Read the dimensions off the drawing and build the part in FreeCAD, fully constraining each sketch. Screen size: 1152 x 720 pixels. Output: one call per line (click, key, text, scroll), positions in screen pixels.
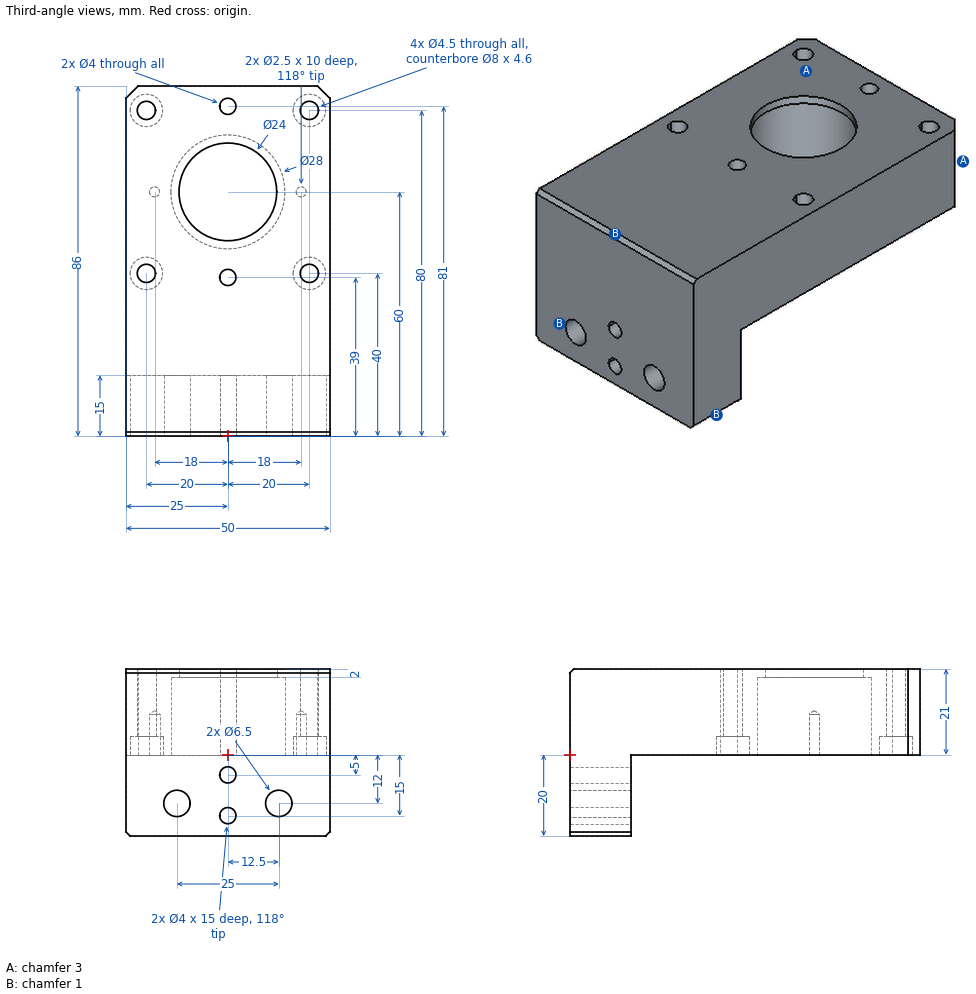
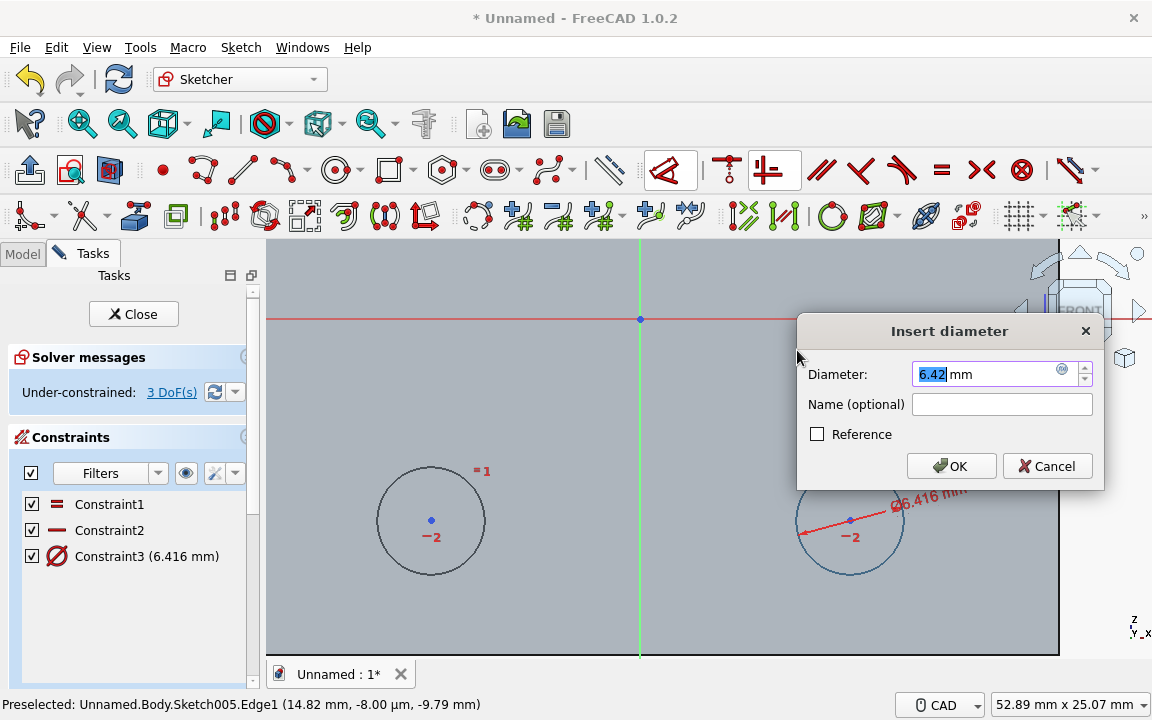
text(6.5)
key(Return)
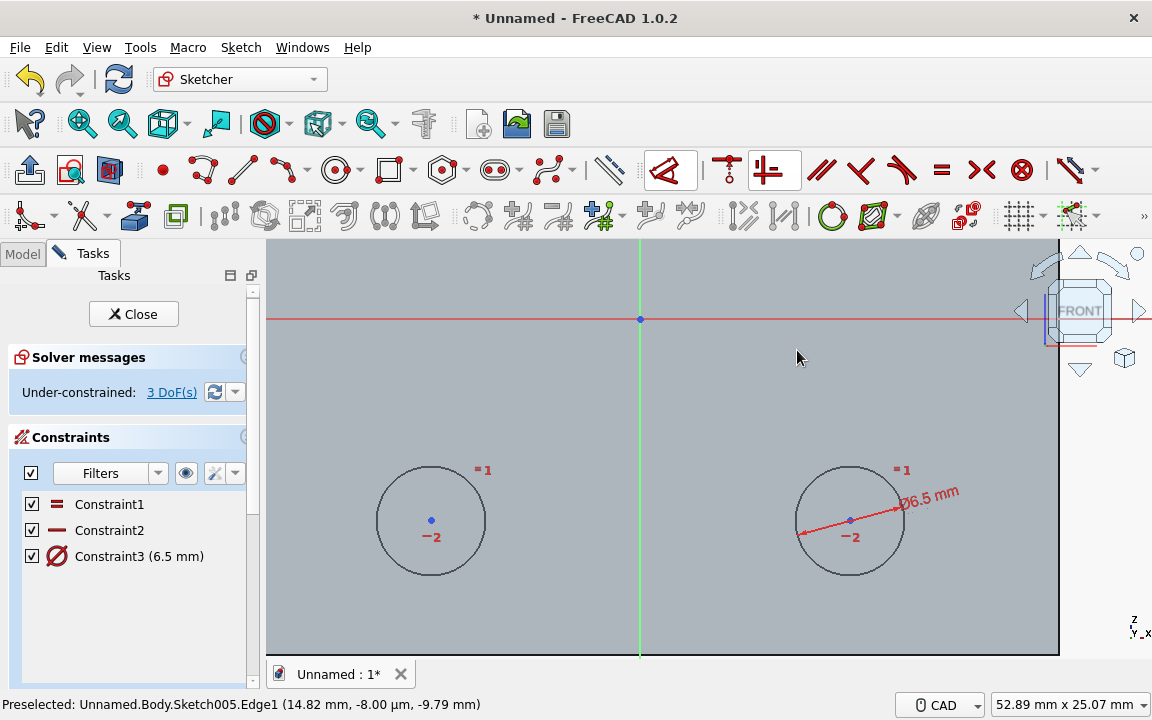
click(850, 521)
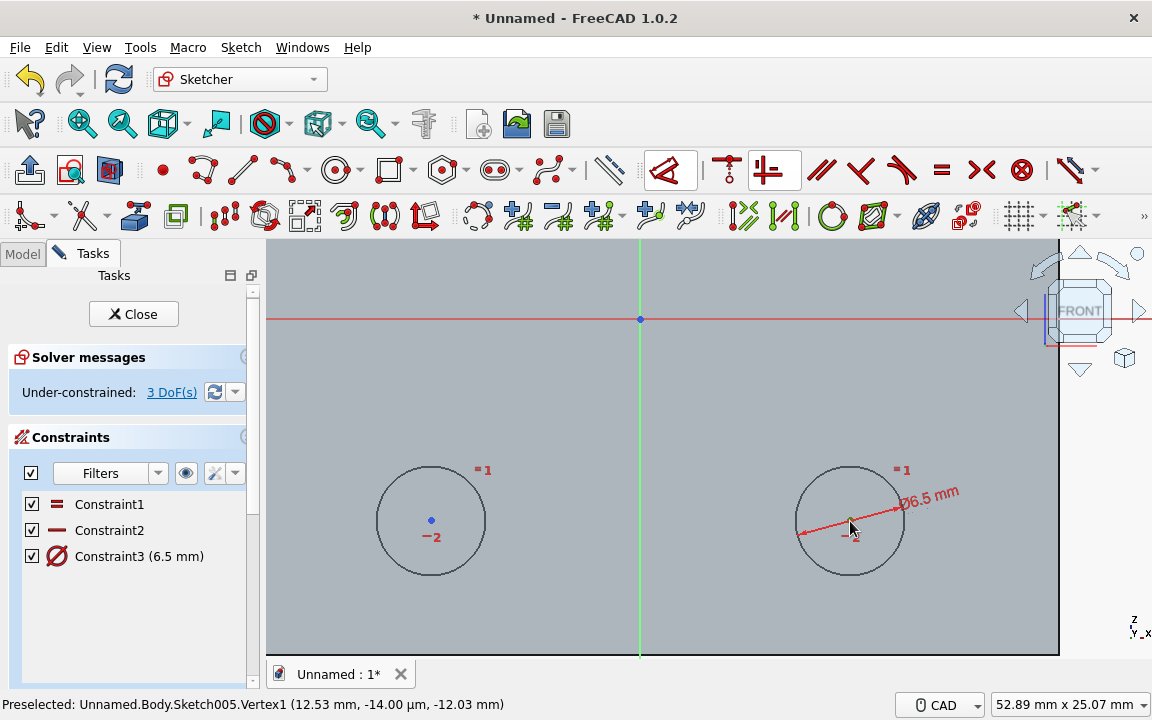
click(692, 170)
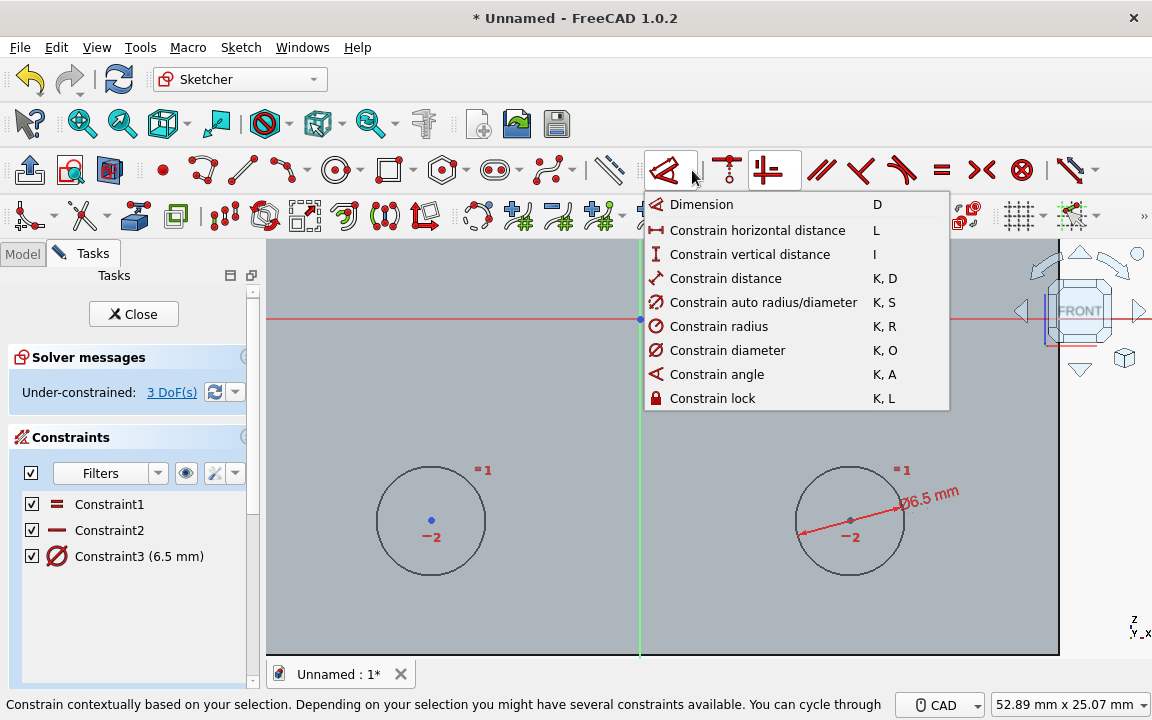
click(797, 254)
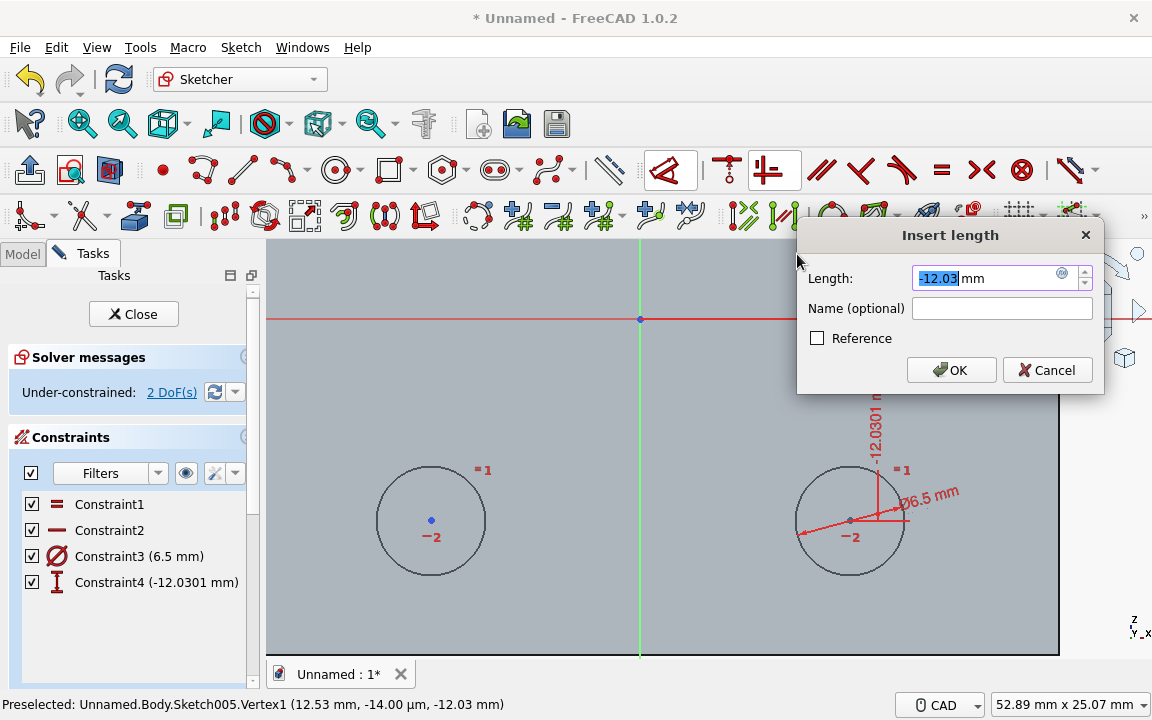
text(-12)
key(Return)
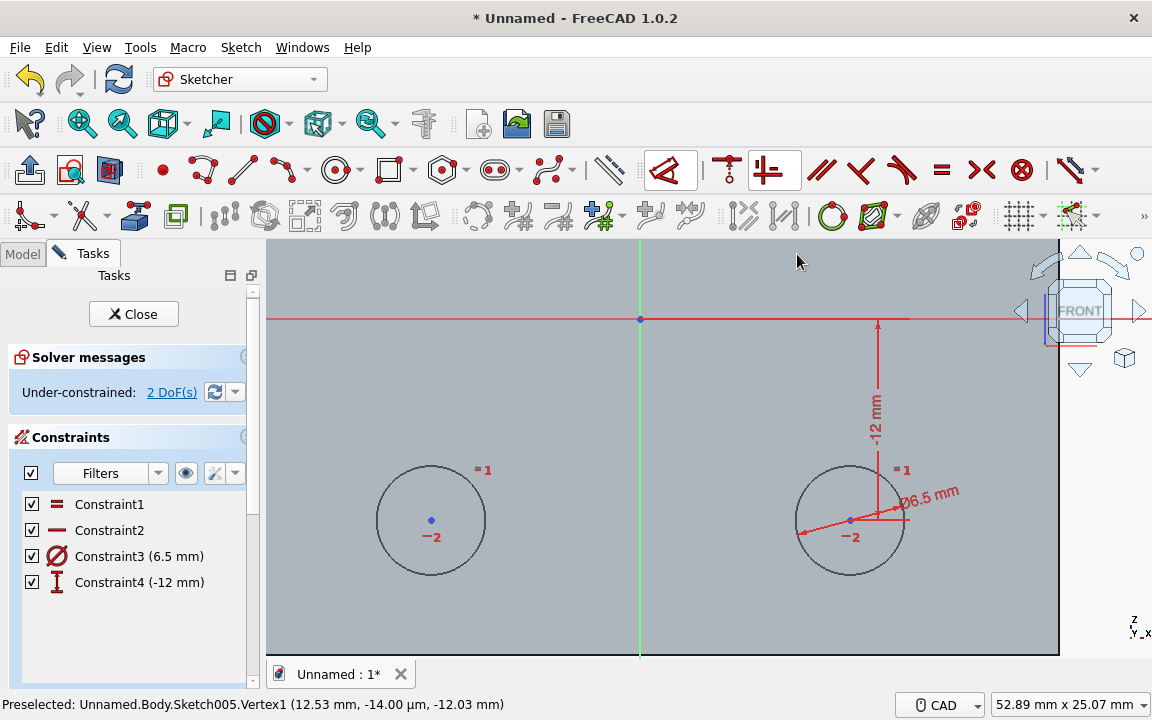
click(850, 520)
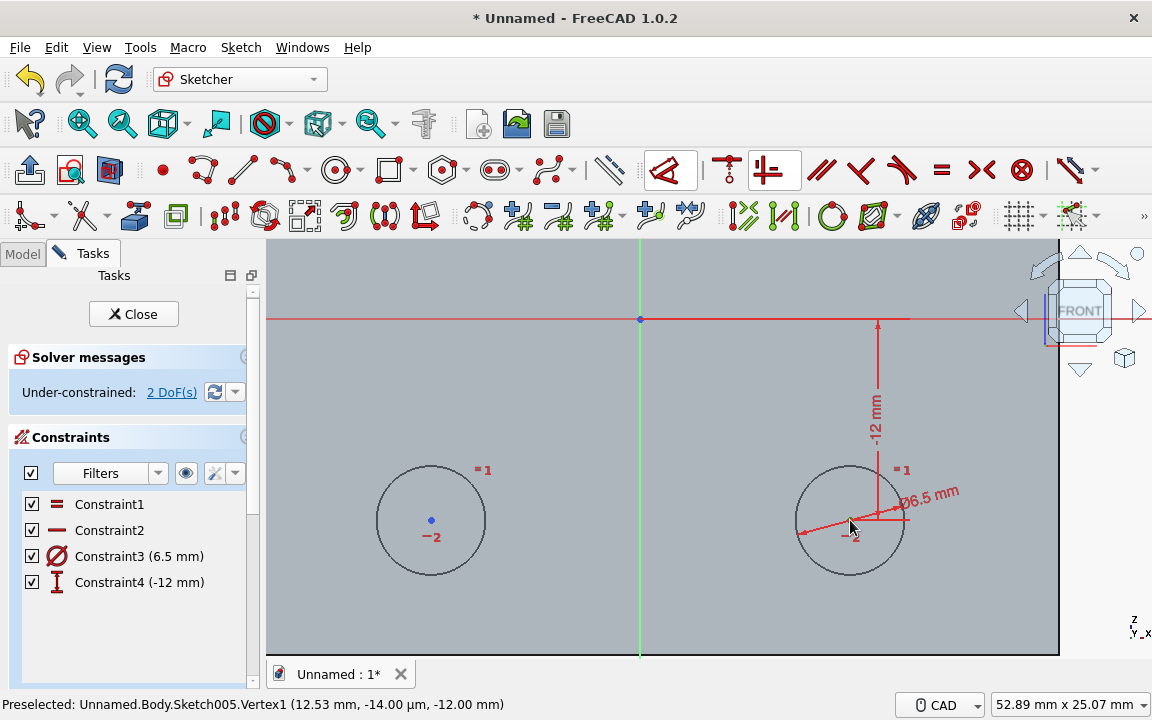
click(431, 520)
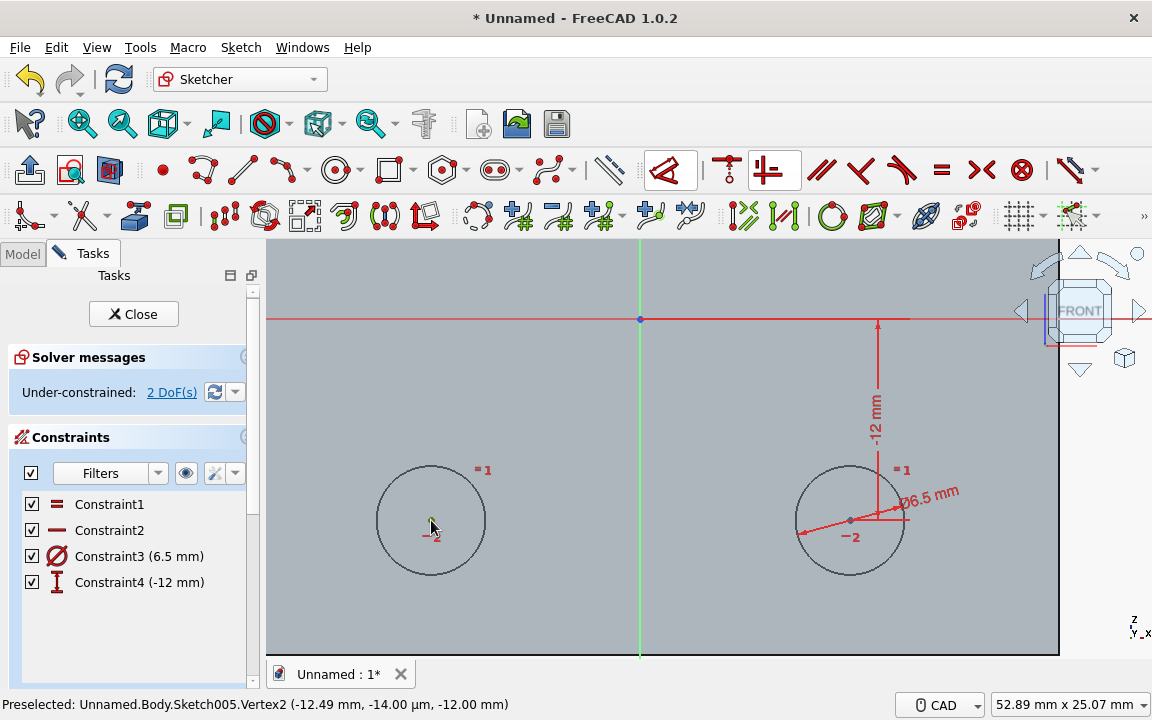
key(l)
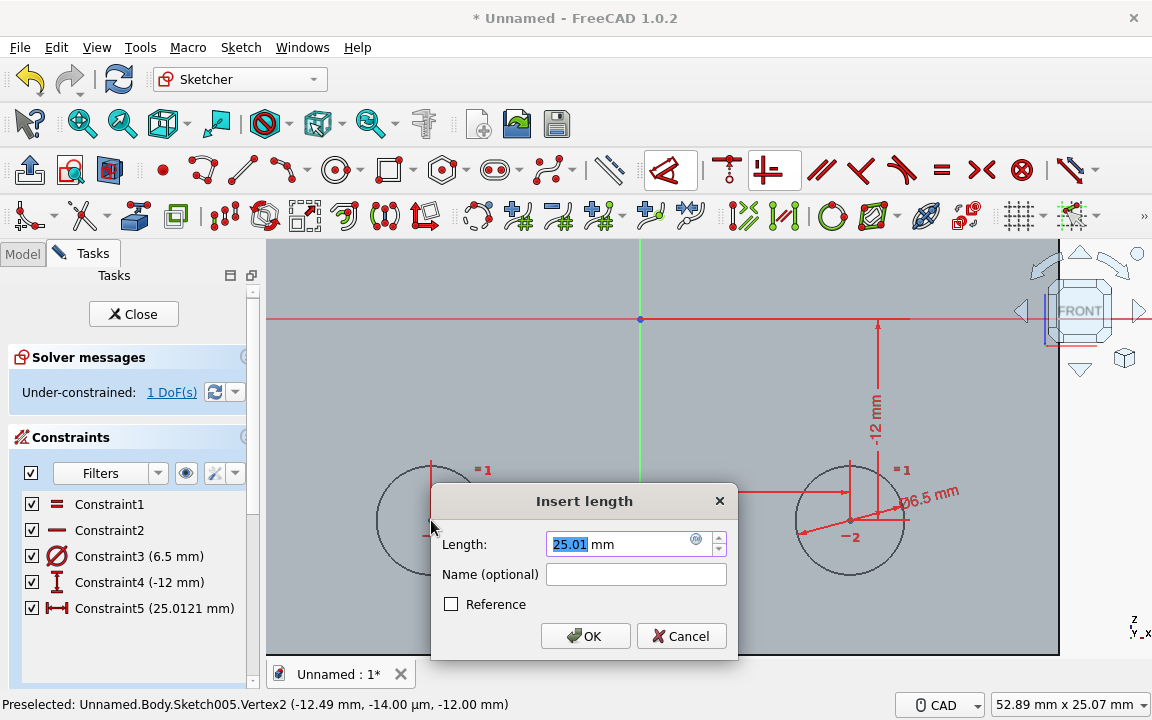
text(25)
key(Return)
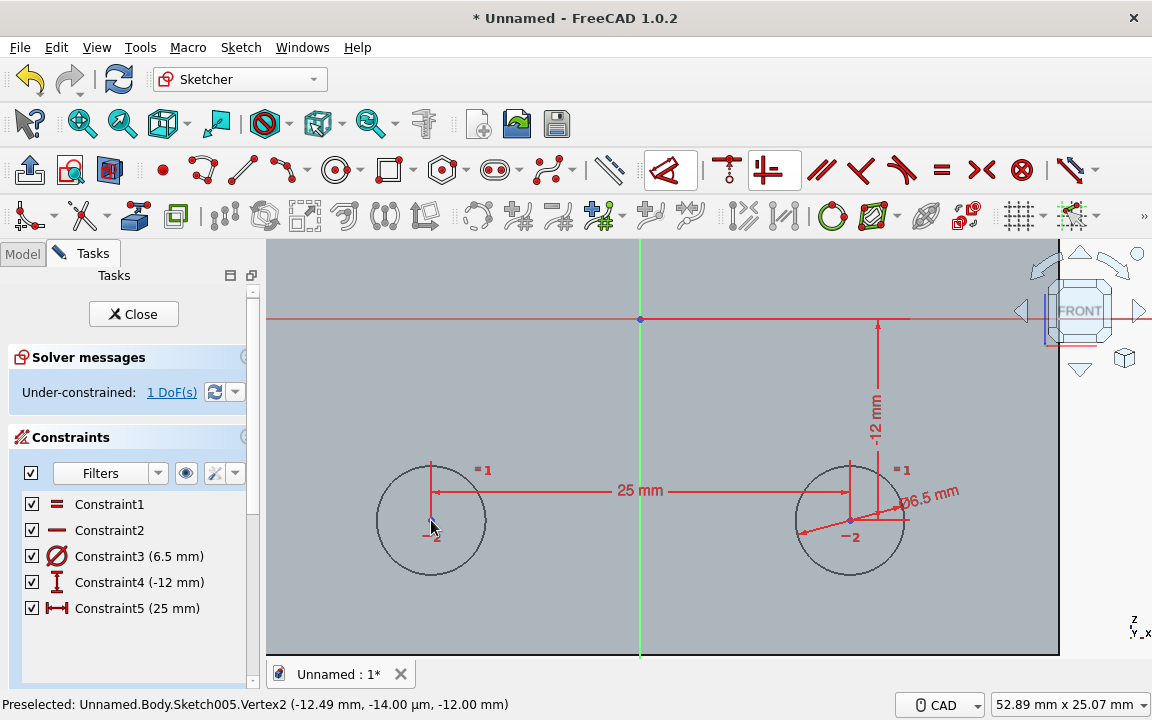
click(850, 520)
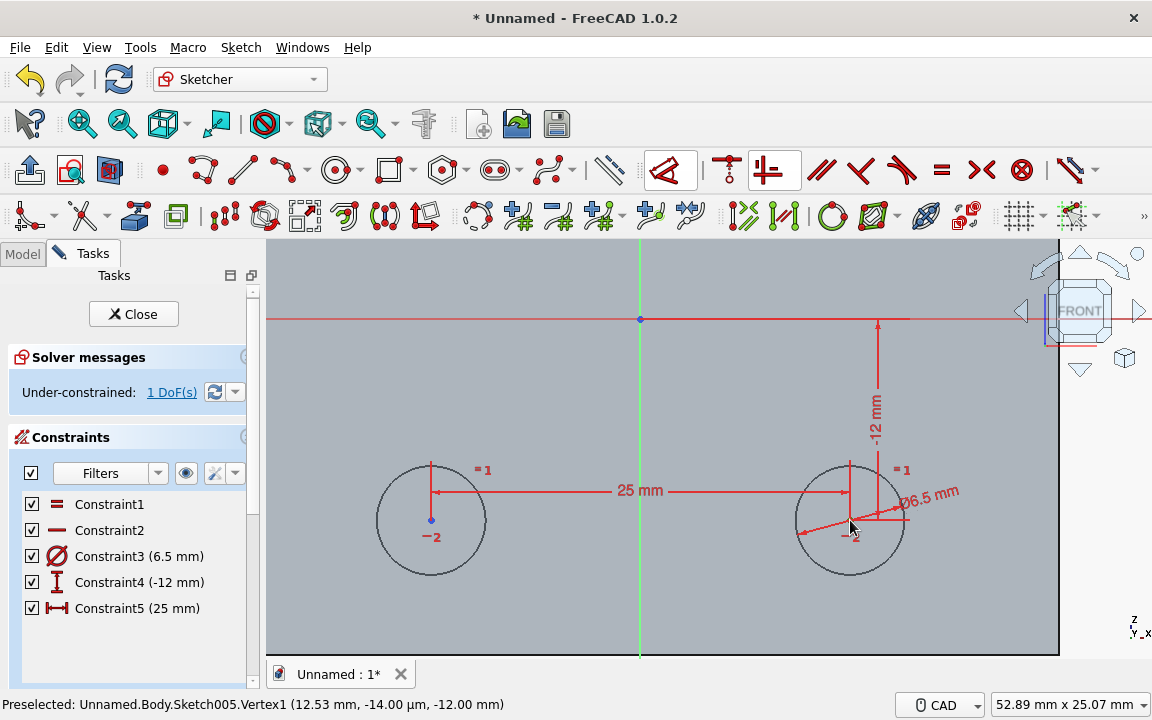
click(692, 170)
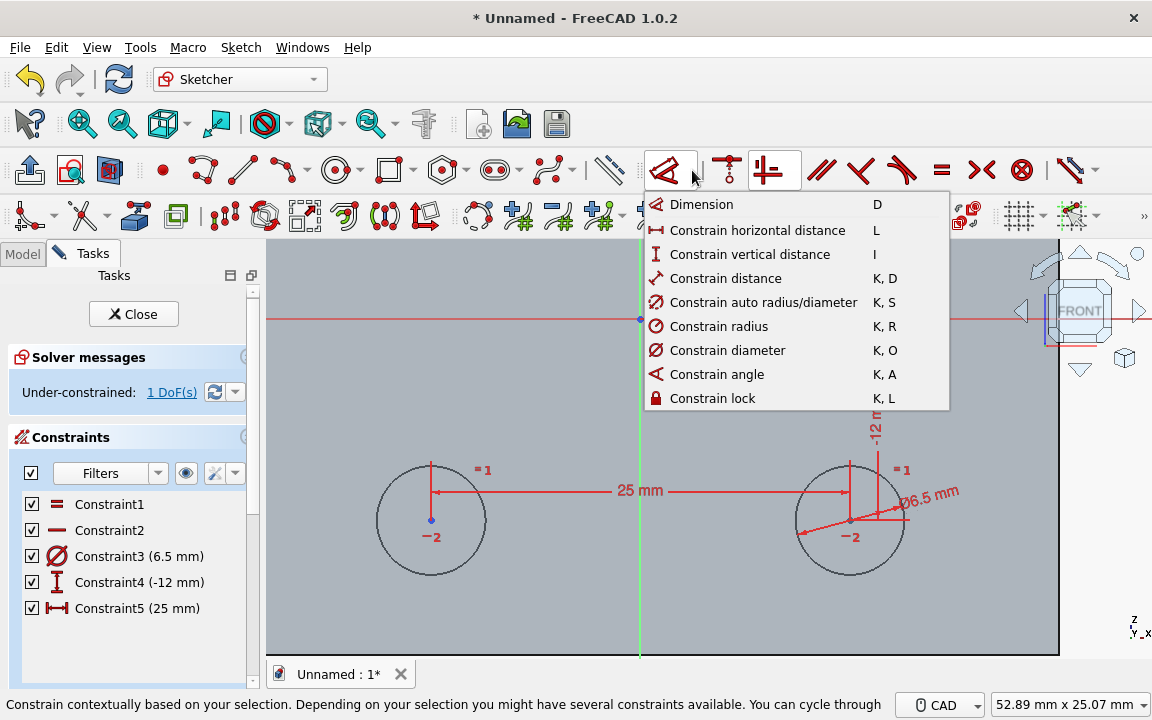
click(797, 230)